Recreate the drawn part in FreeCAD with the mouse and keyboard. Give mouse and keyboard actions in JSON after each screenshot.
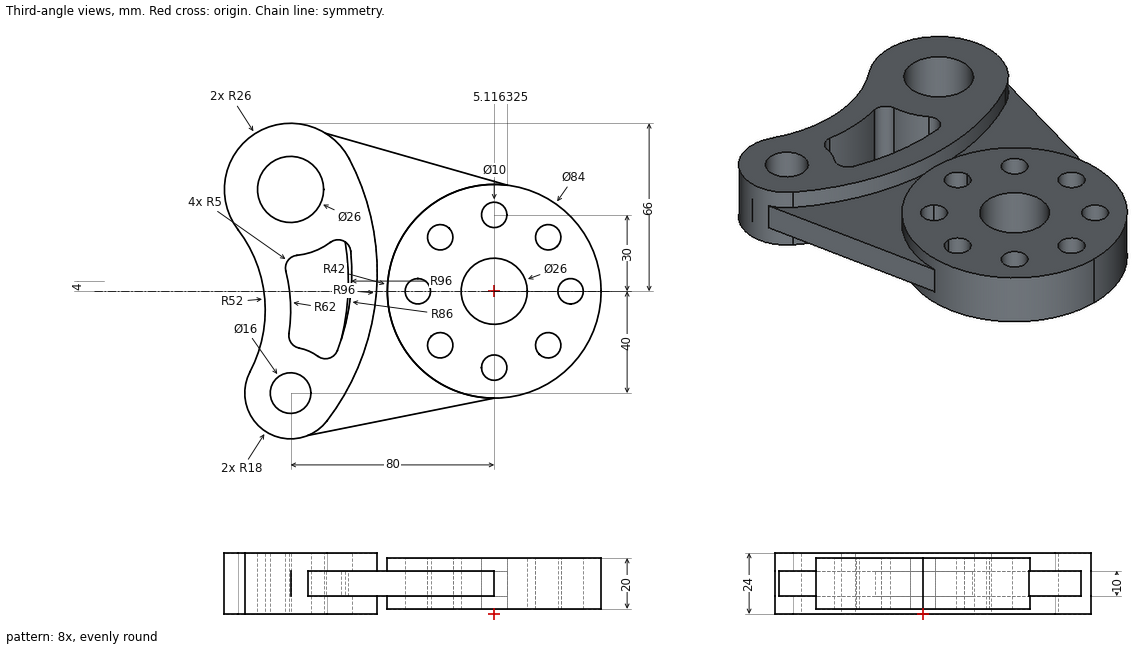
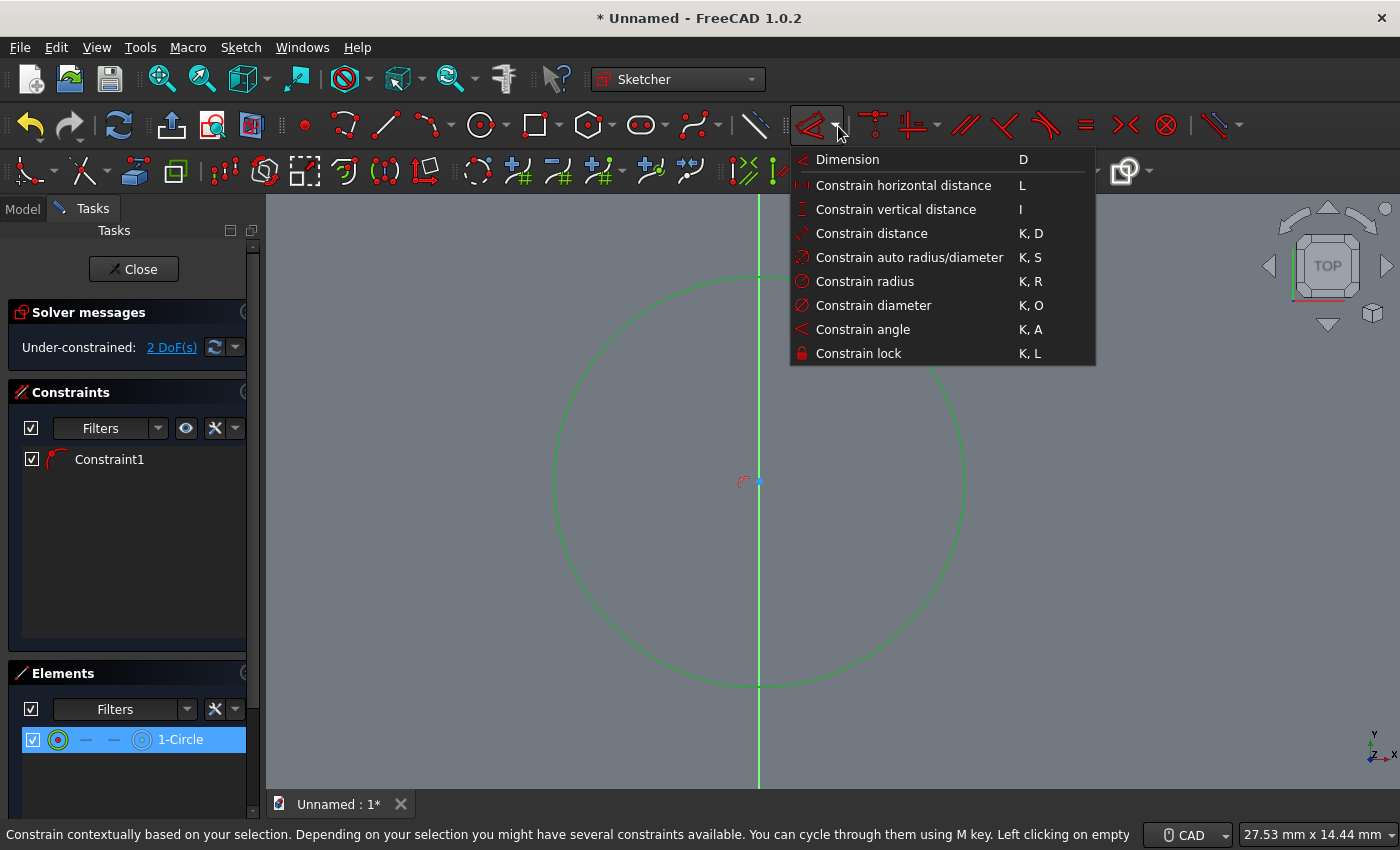
{"action": "left_click", "coordinate": [943, 305]}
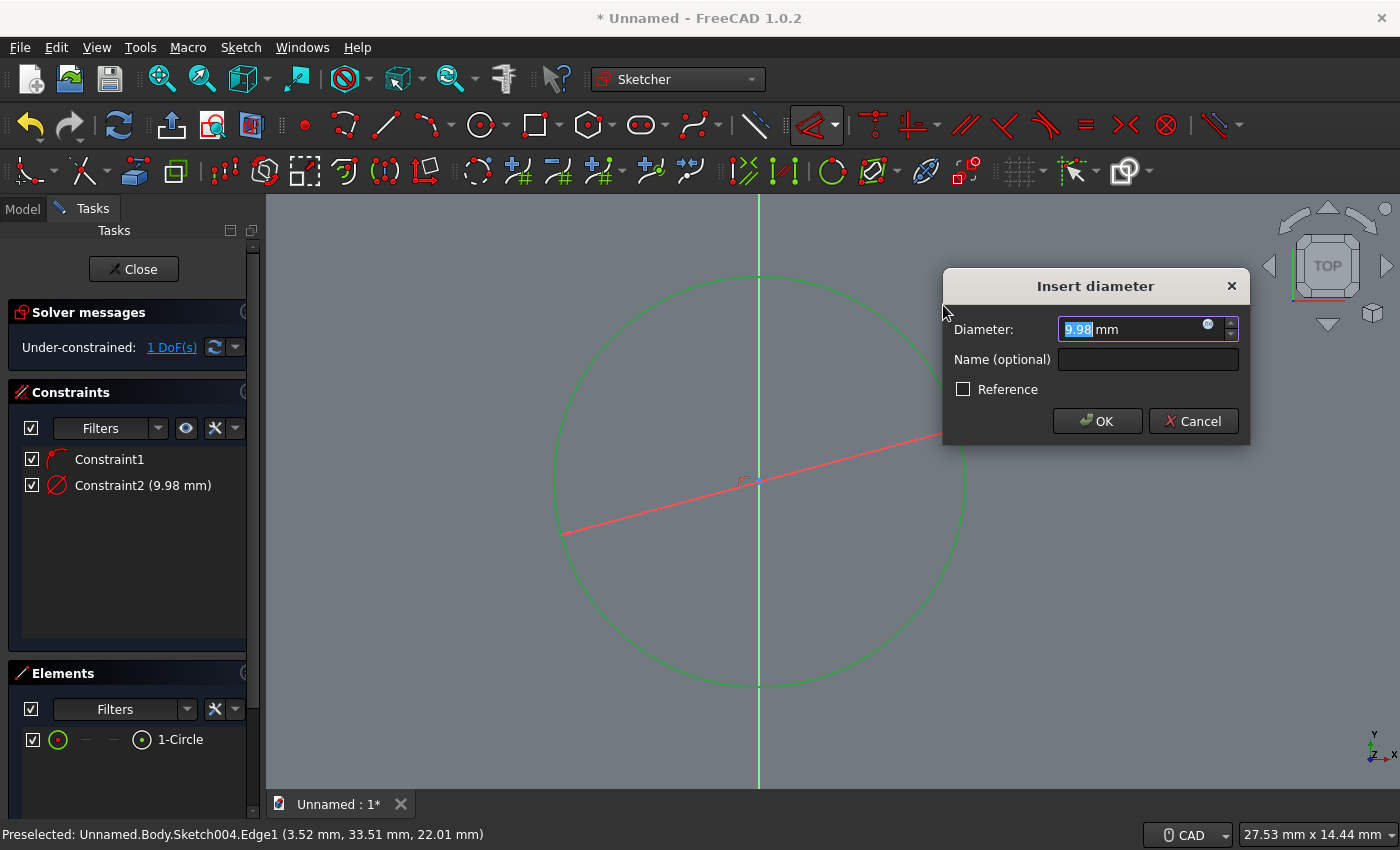
{"action": "type", "text": "10"}
{"action": "key", "text": "Return"}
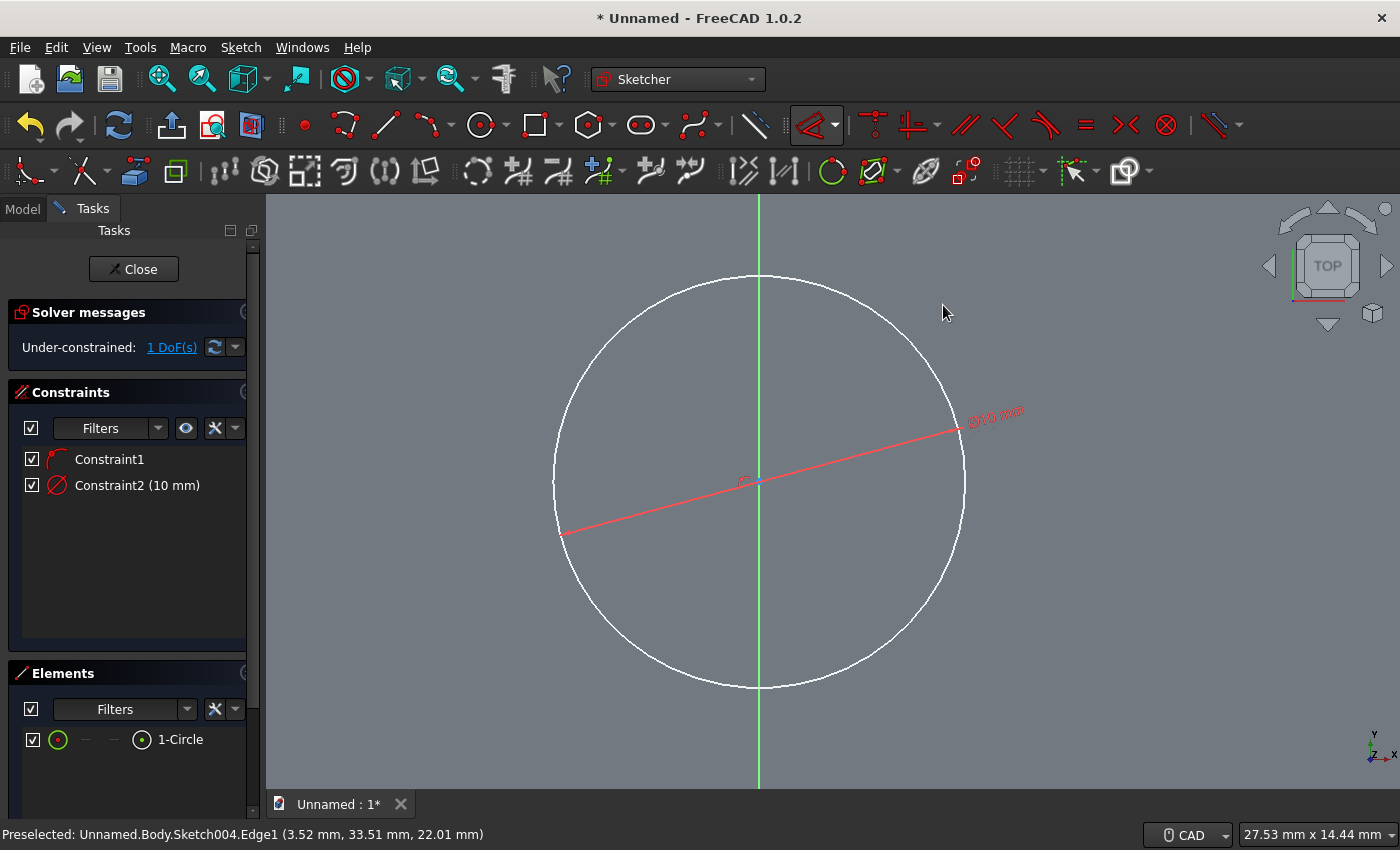
{"action": "left_click", "coordinate": [759, 482]}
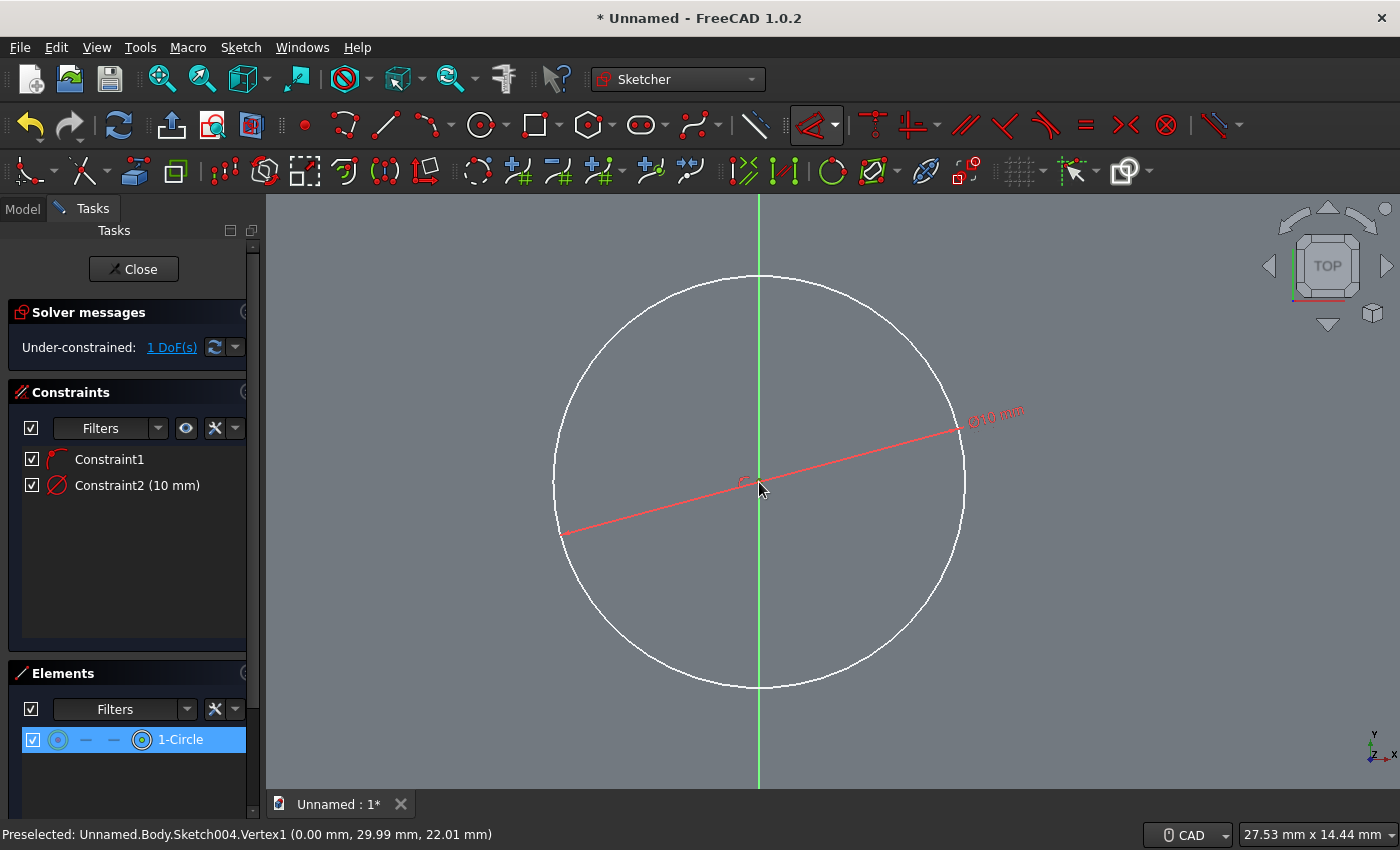
{"action": "left_click", "coordinate": [838, 126]}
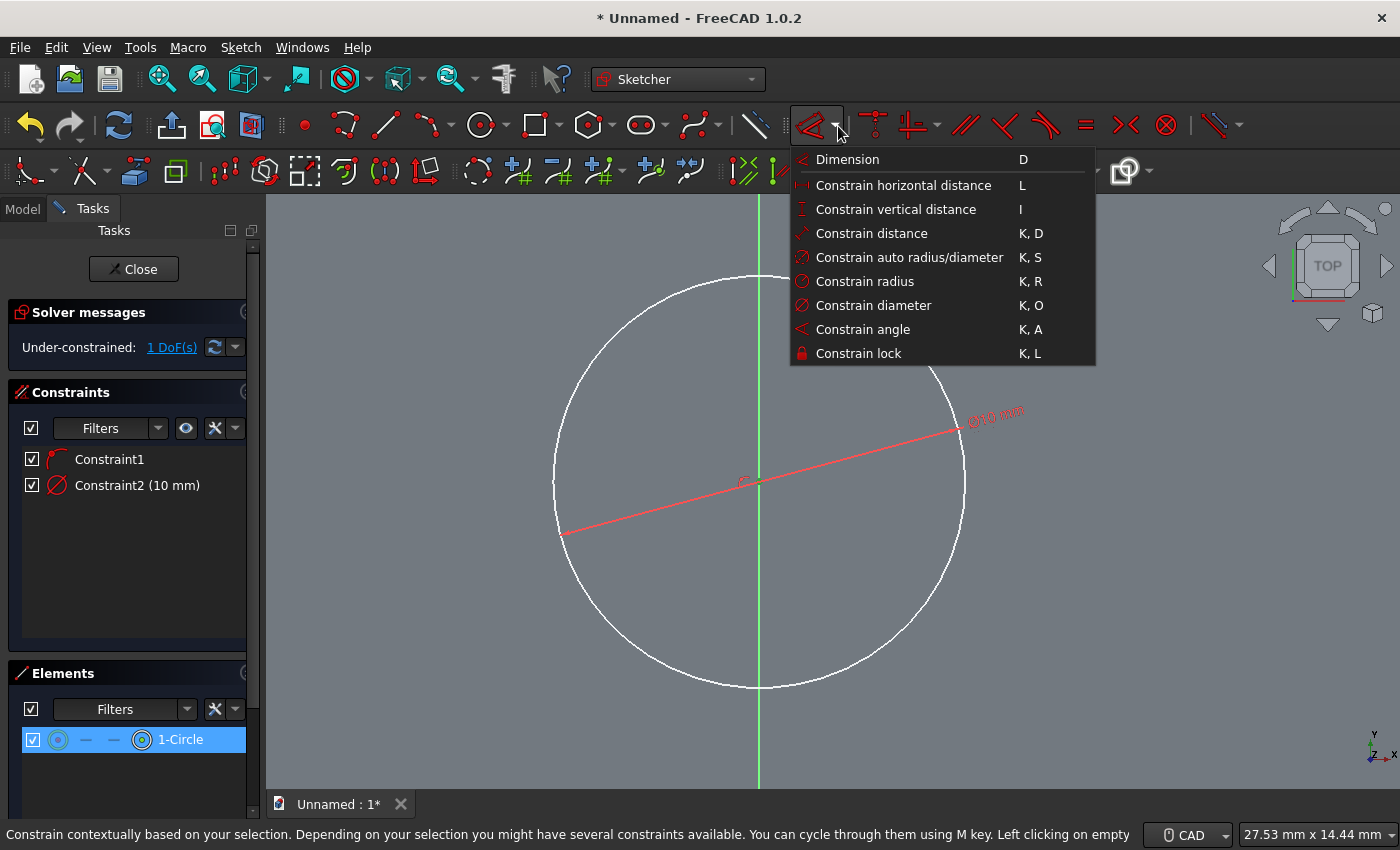
{"action": "left_click", "coordinate": [943, 209]}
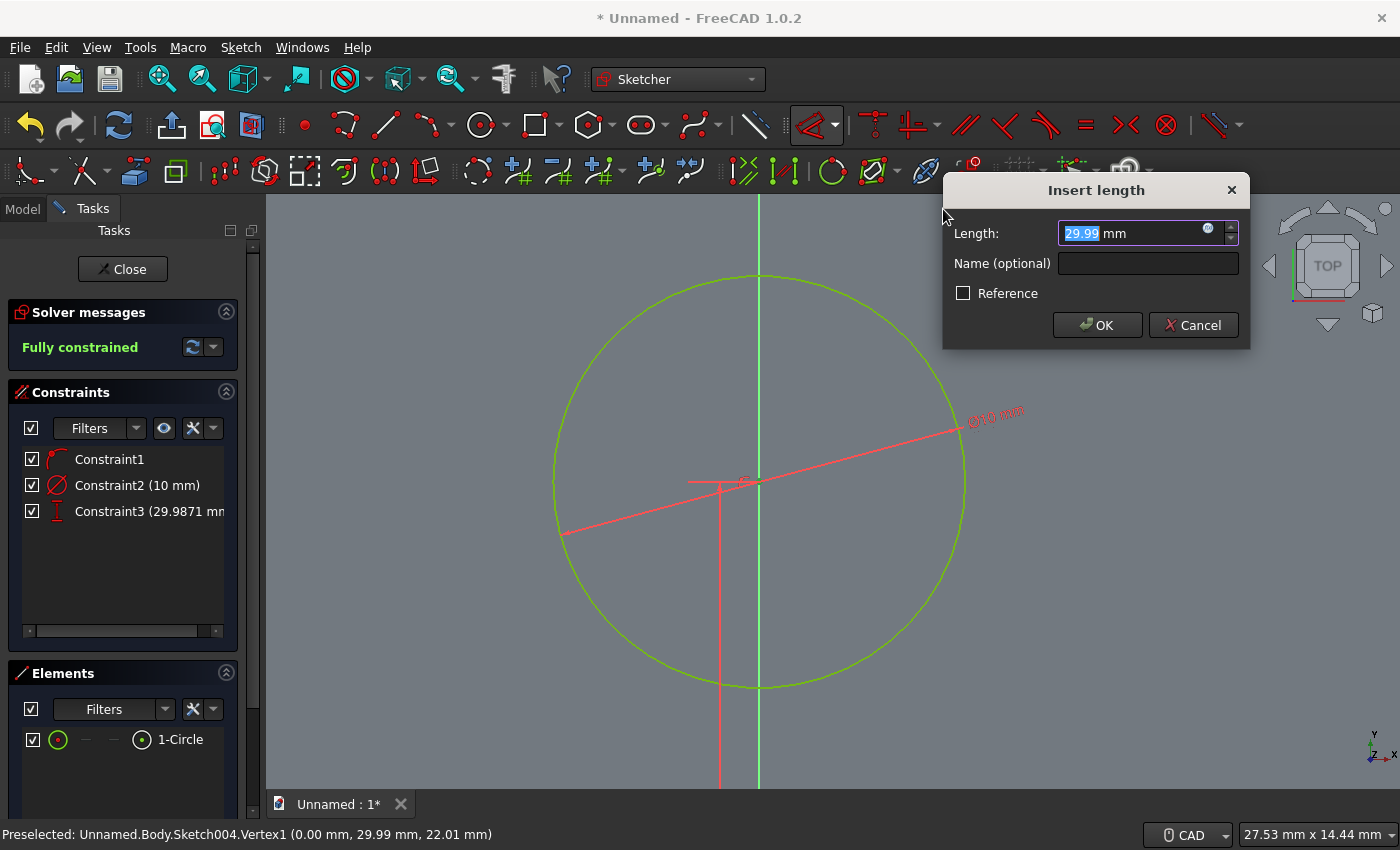
{"action": "type", "text": "30"}
{"action": "key", "text": "Return"}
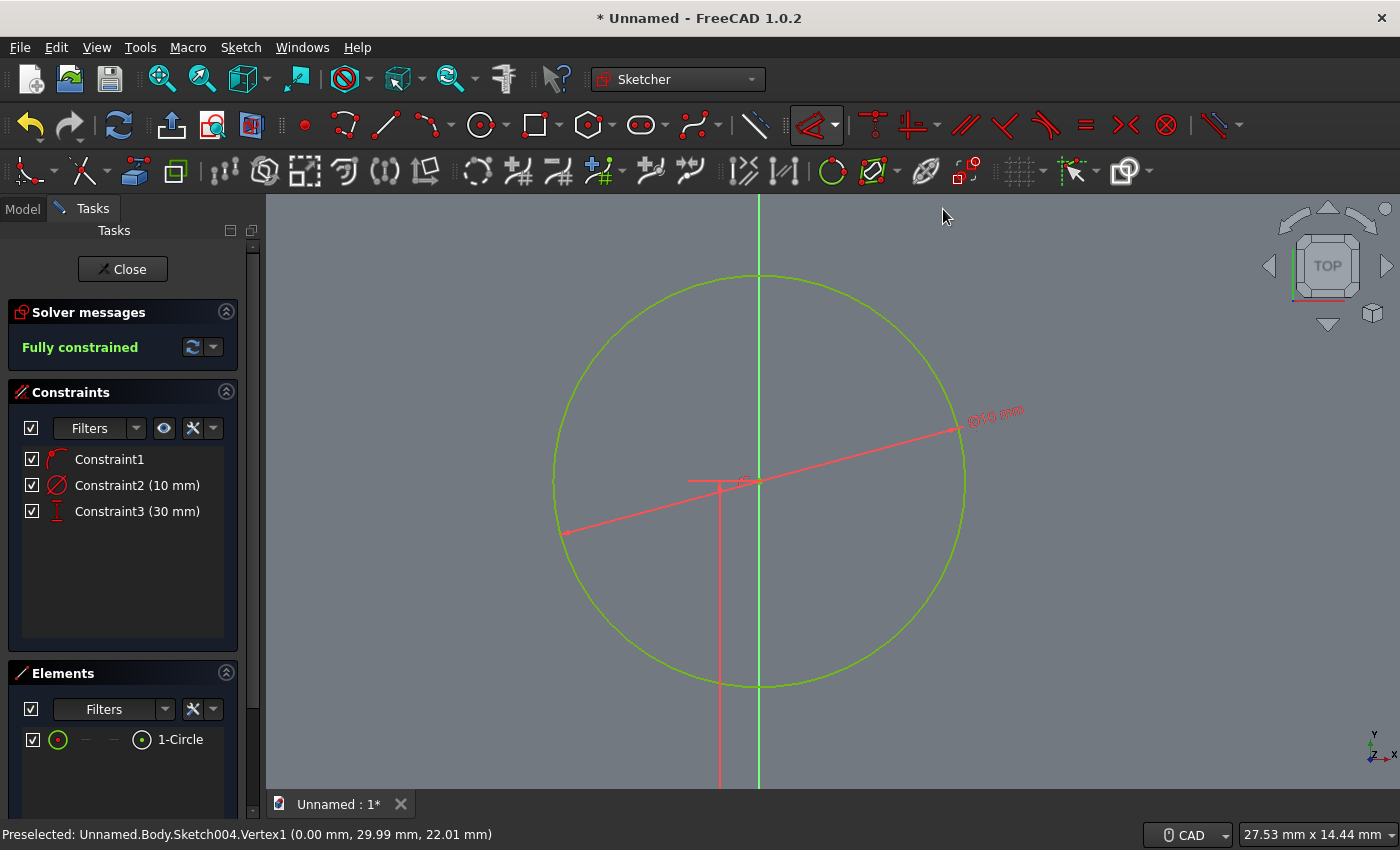
{"action": "left_click", "coordinate": [123, 269]}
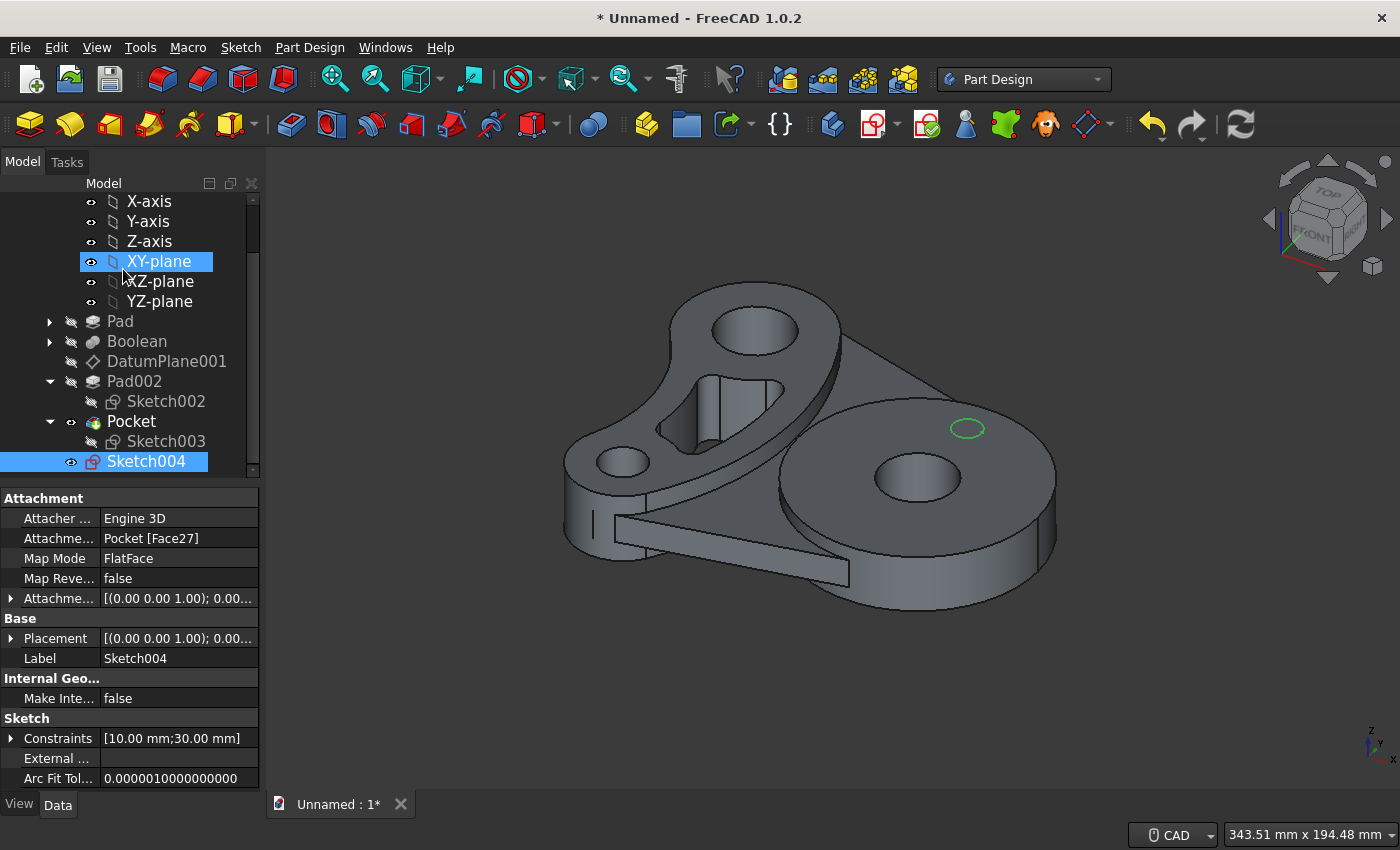
{"action": "left_click", "coordinate": [292, 124]}